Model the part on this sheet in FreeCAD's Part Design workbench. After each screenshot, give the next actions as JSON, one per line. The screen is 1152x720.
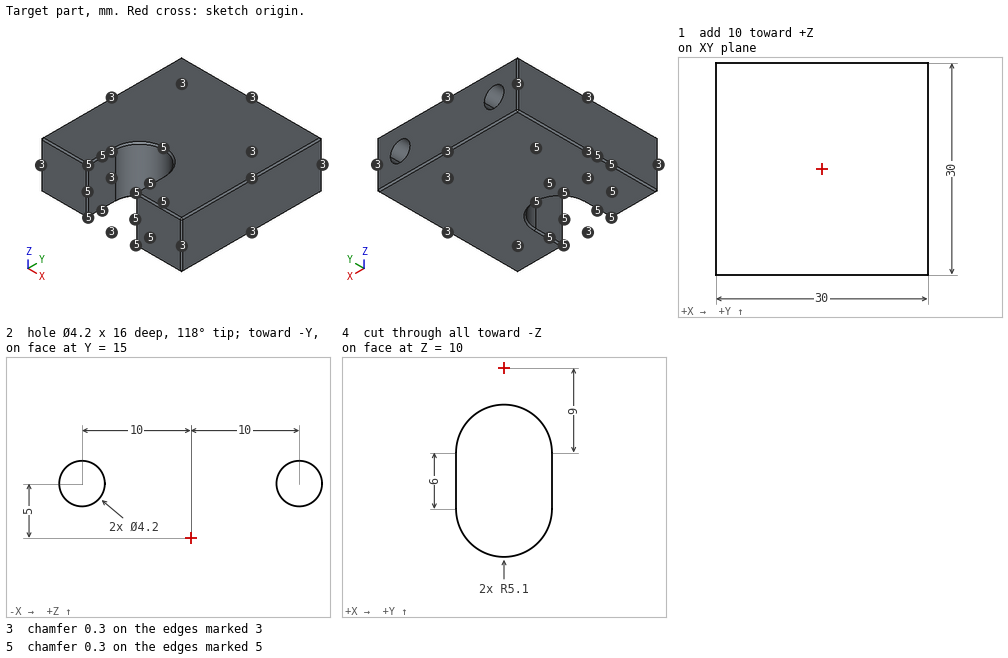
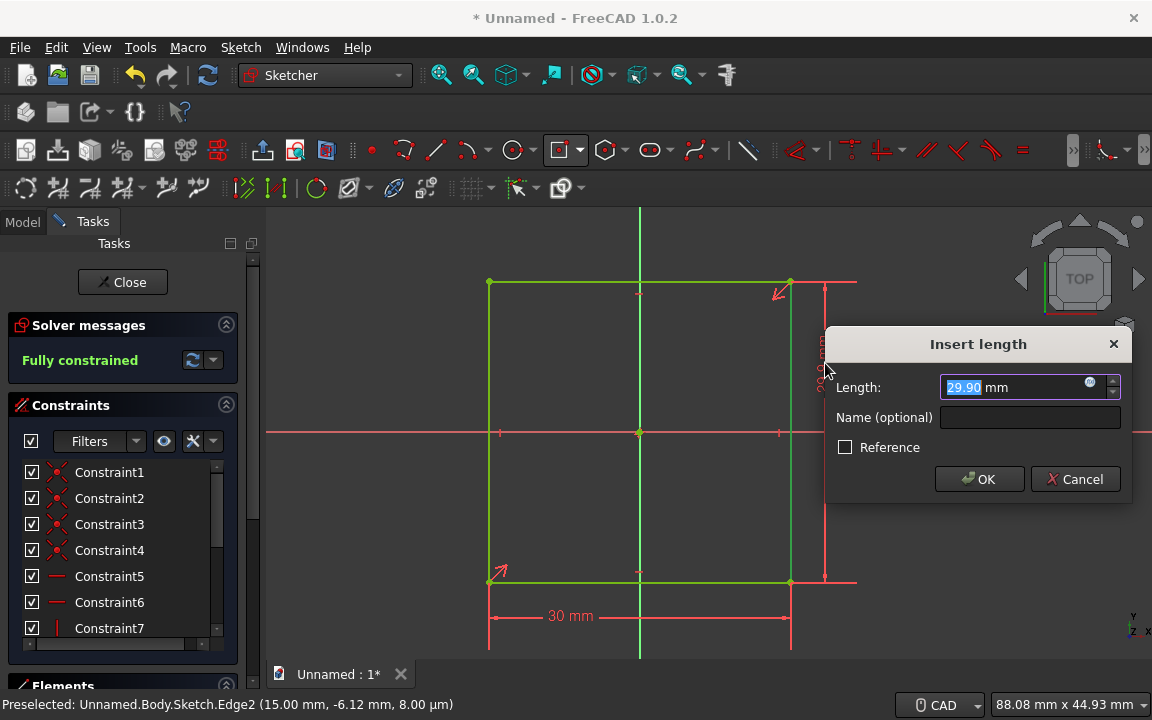
{"action": "type", "text": "30"}
{"action": "key", "text": "Return"}
{"action": "key", "text": "Escape"}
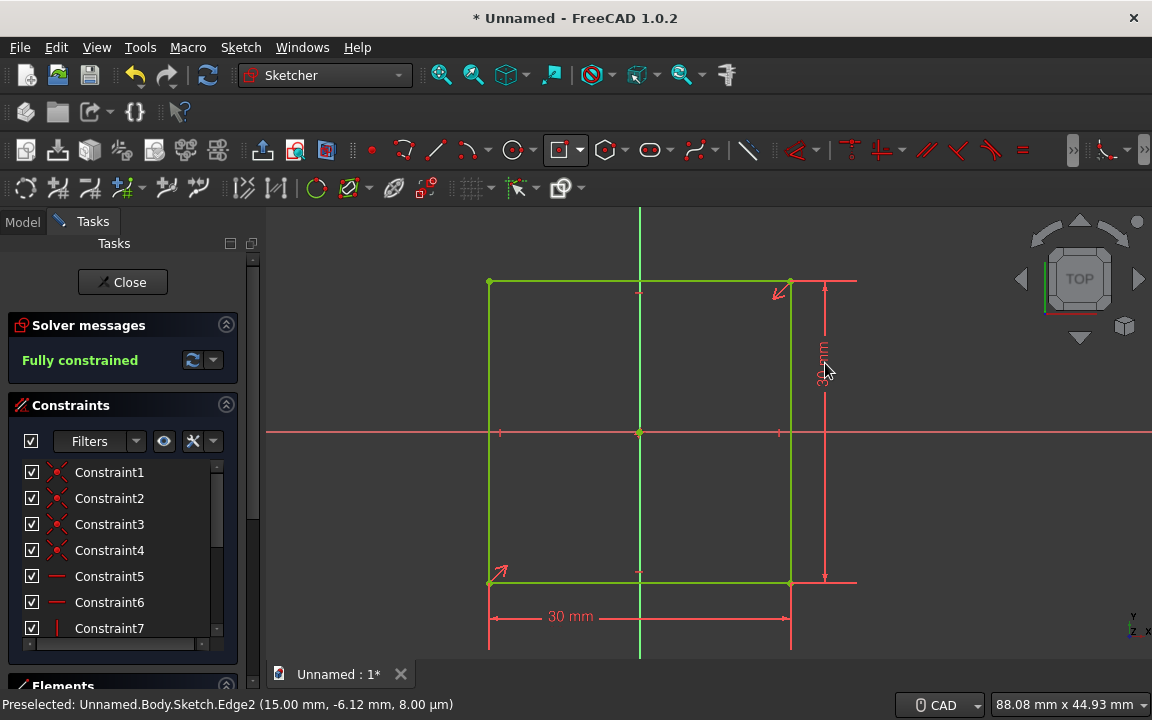
{"action": "left_click", "coordinate": [123, 282]}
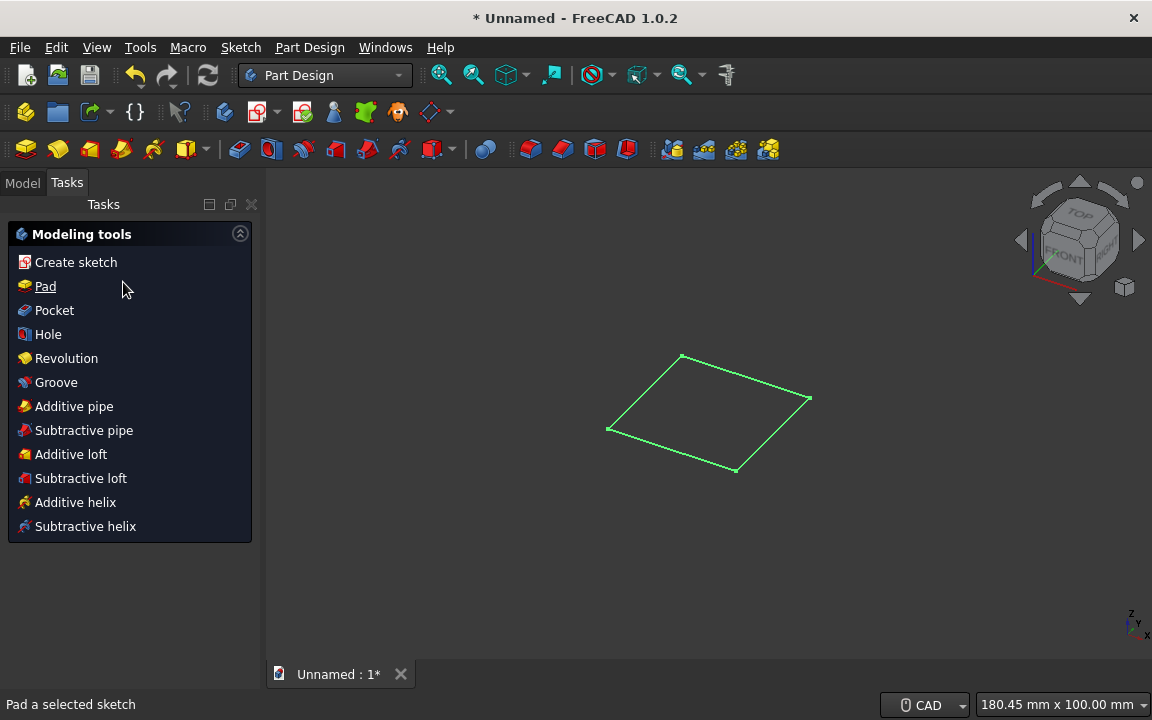
{"action": "left_click", "coordinate": [26, 150]}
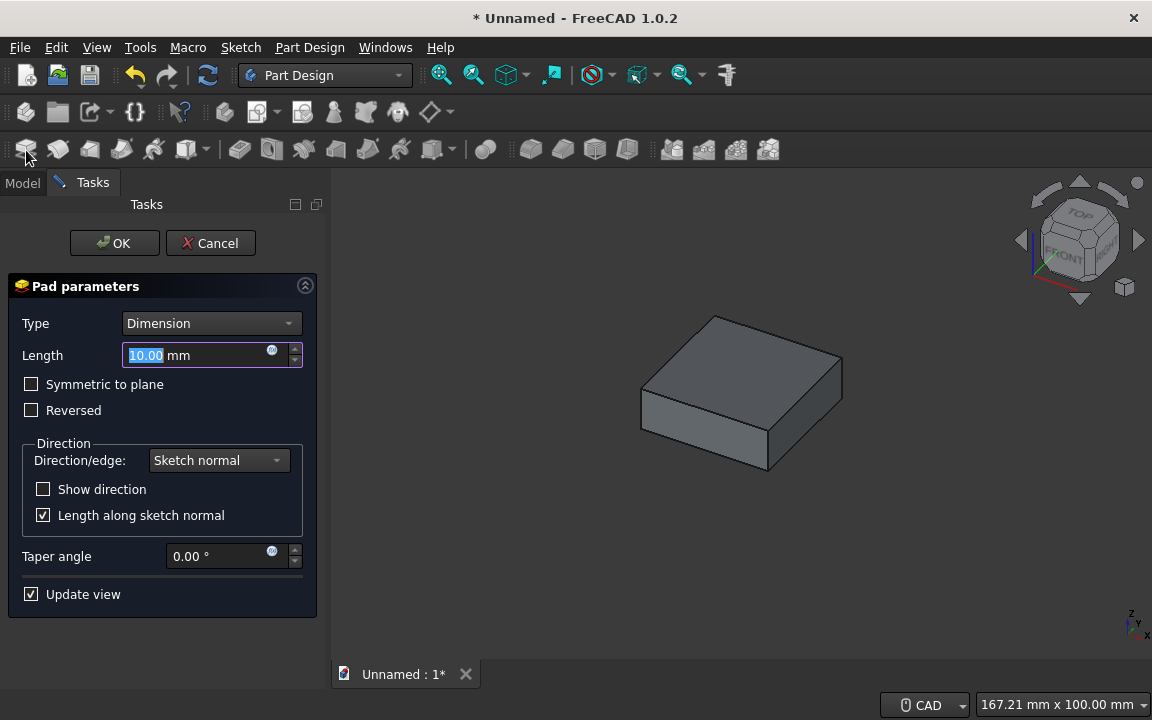
{"action": "type", "text": "10"}
{"action": "key", "text": "Tab"}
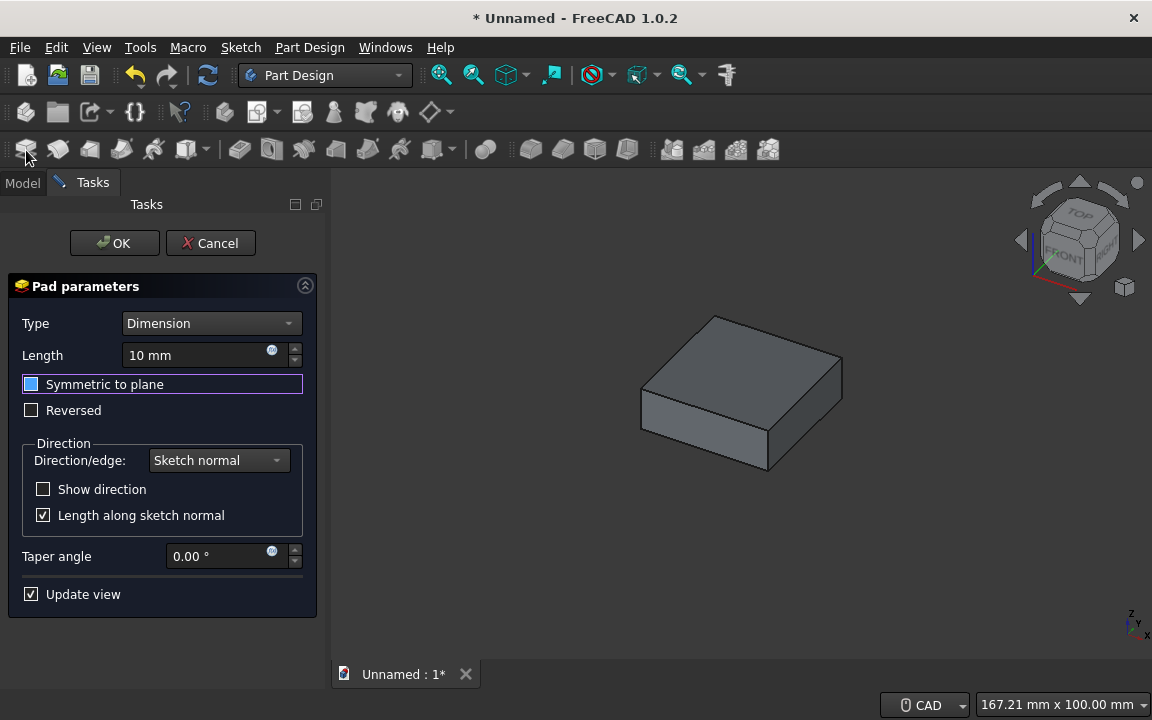
{"action": "left_click", "coordinate": [115, 243]}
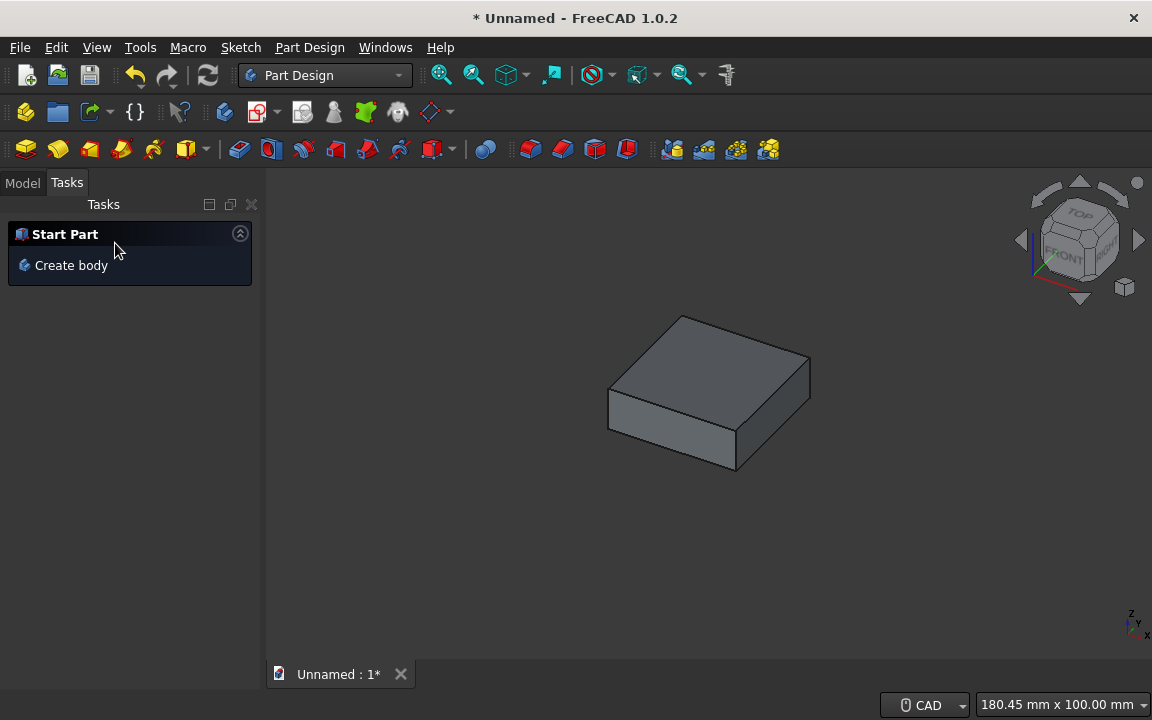
{"action": "left_click", "coordinate": [442, 76]}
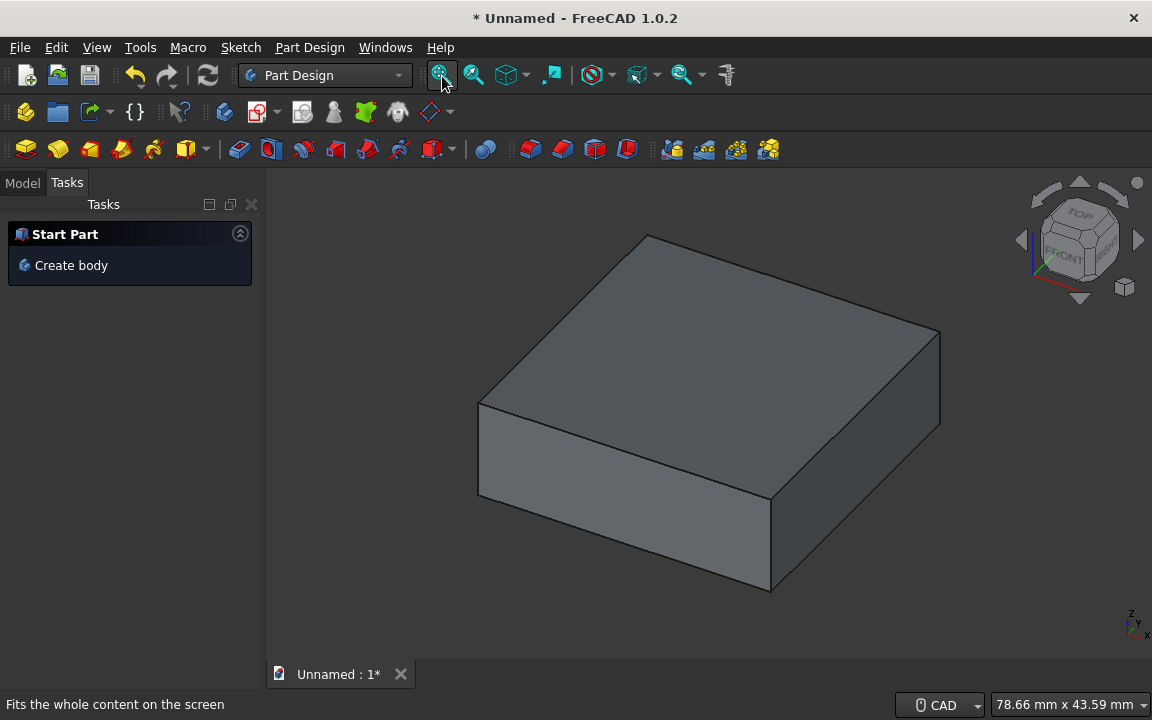
{"action": "key", "text": "4"}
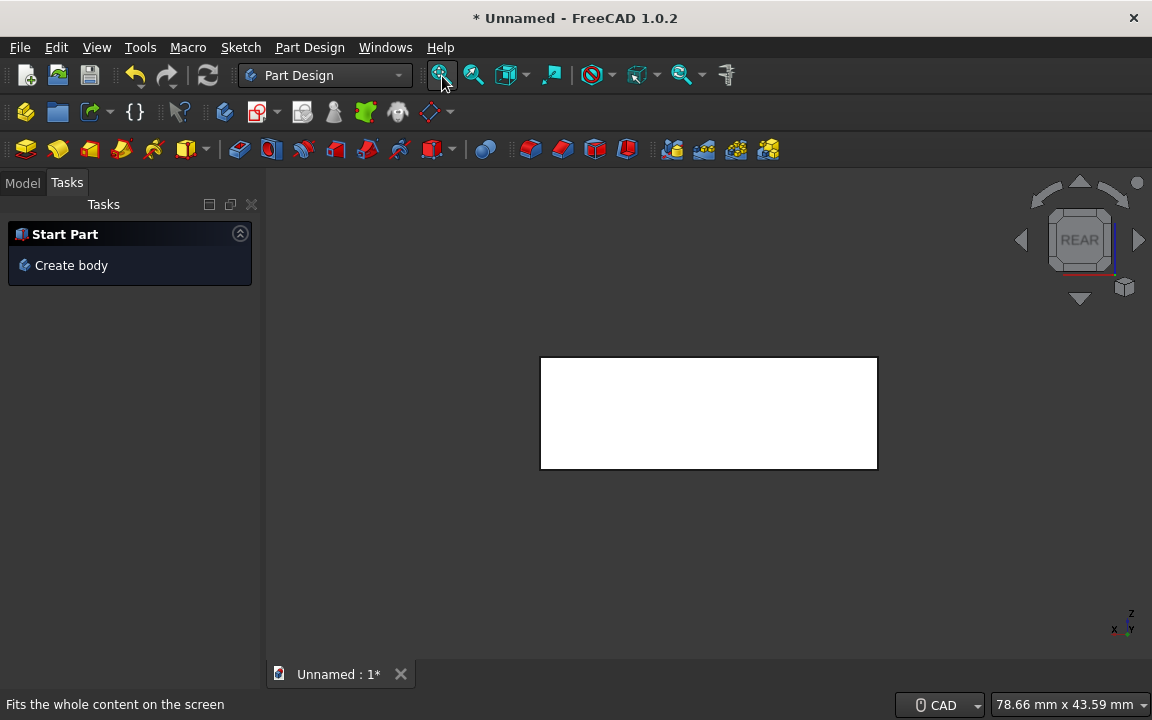
{"action": "left_click", "coordinate": [442, 76]}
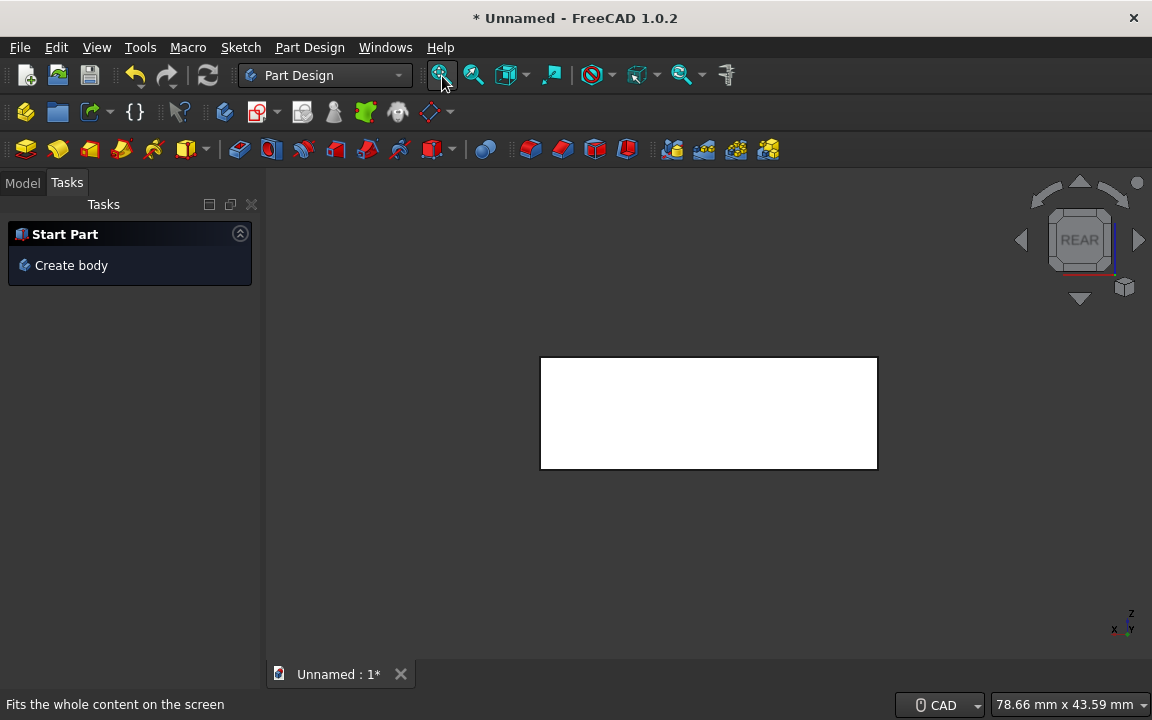
{"action": "left_click", "coordinate": [612, 413]}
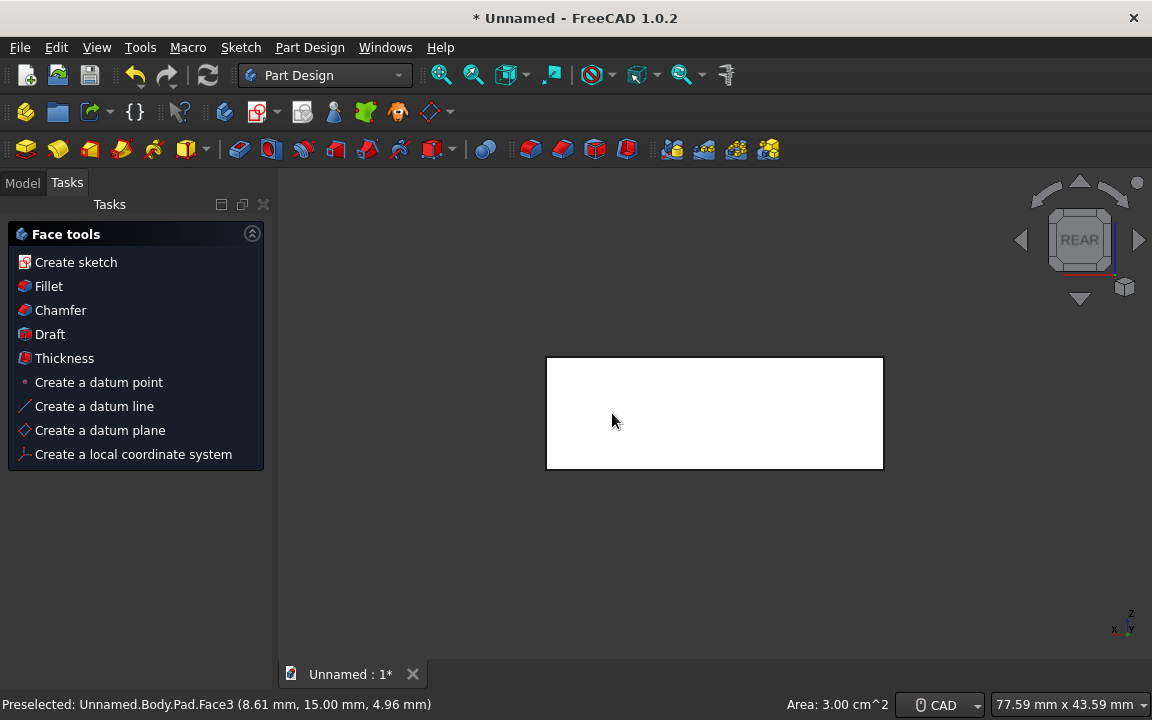
{"action": "left_click", "coordinate": [258, 112]}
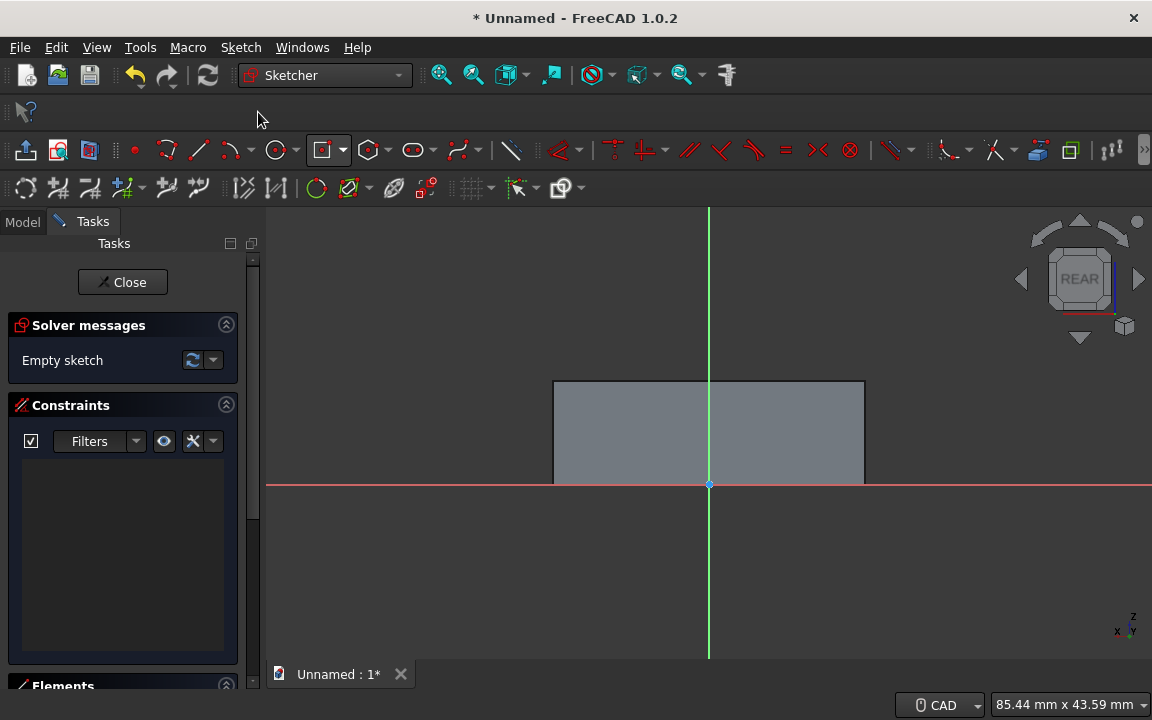
{"action": "scroll", "coordinate": [792, 466], "scroll_direction": "up", "scroll_amount": 3}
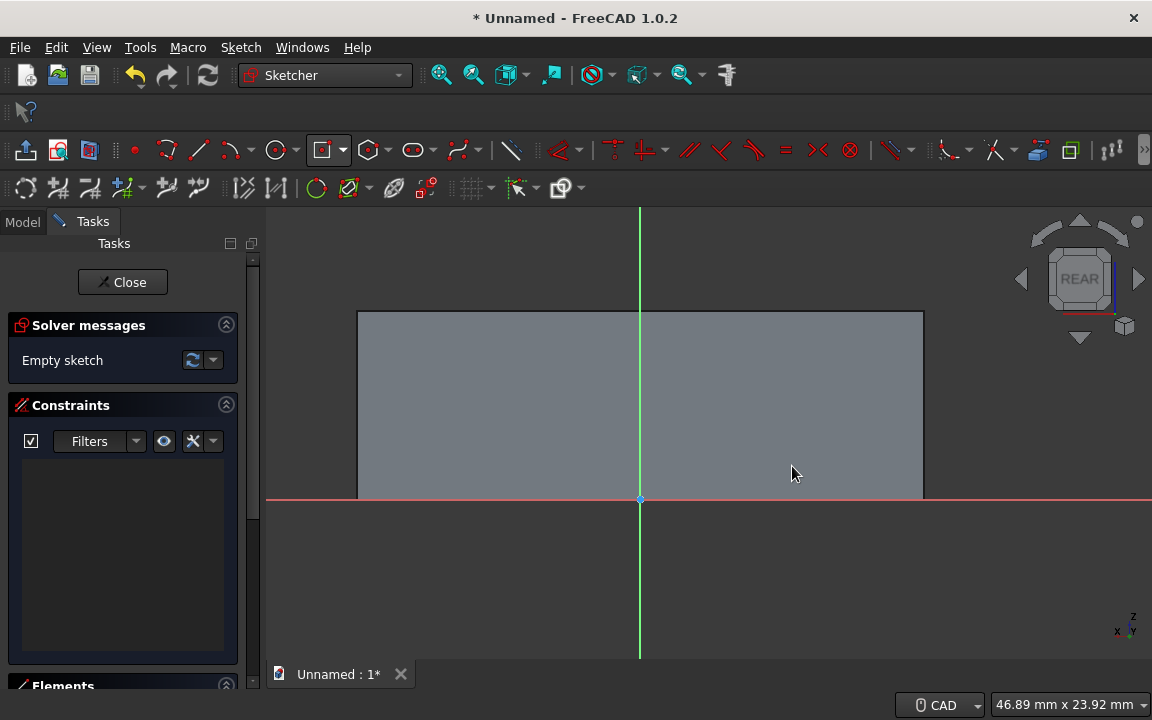
{"action": "left_click", "coordinate": [276, 150]}